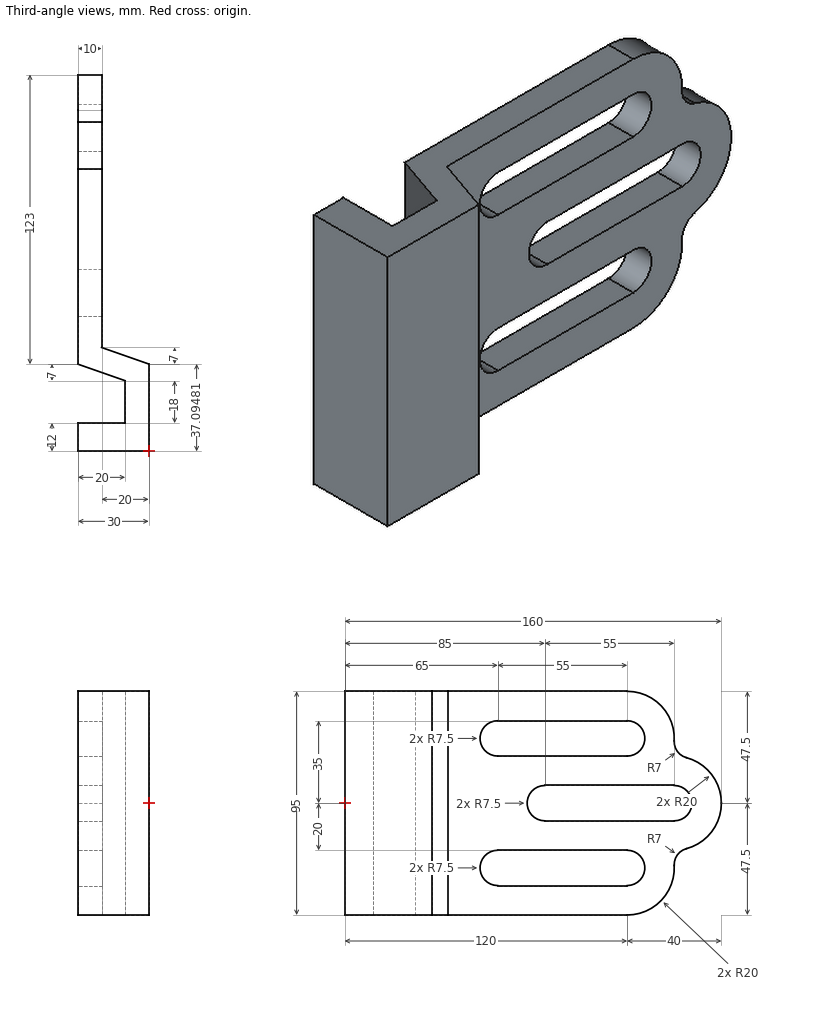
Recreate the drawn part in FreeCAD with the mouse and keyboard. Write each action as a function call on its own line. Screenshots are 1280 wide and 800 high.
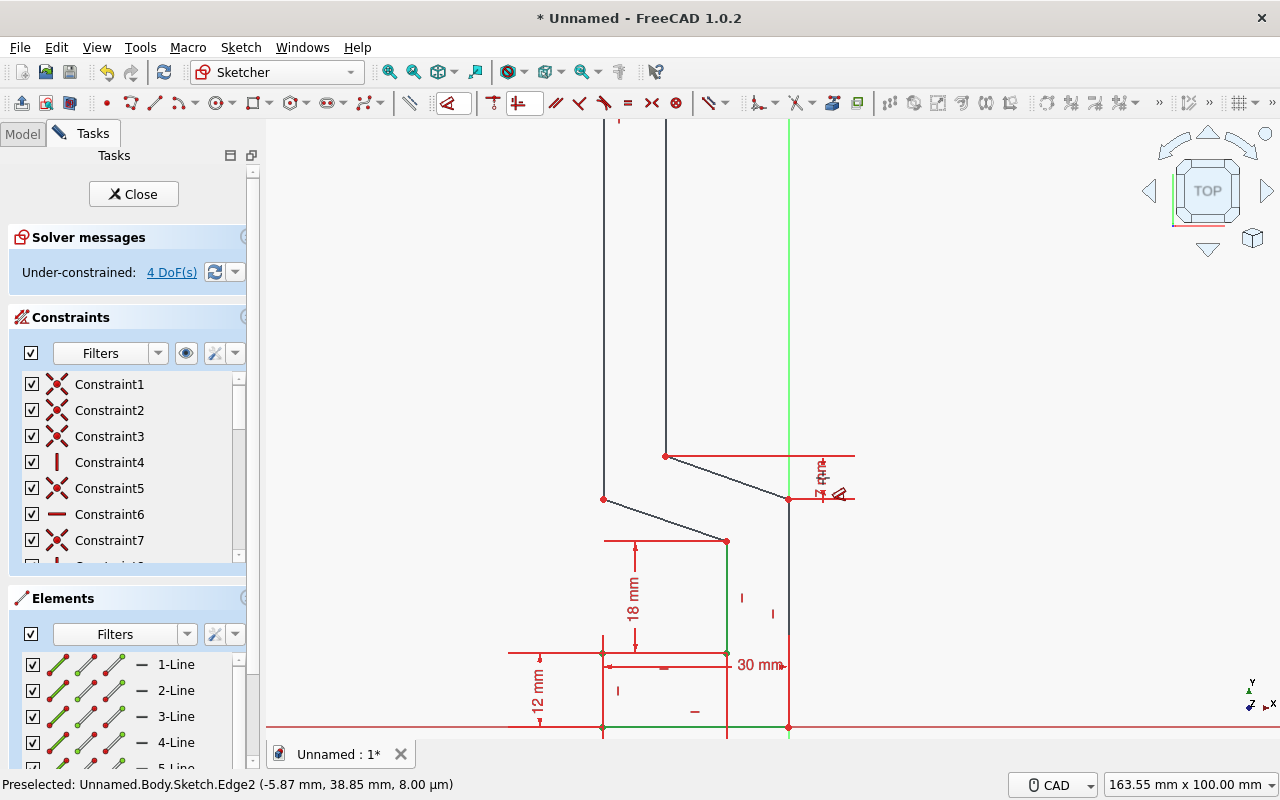
click(641, 512)
click(570, 520)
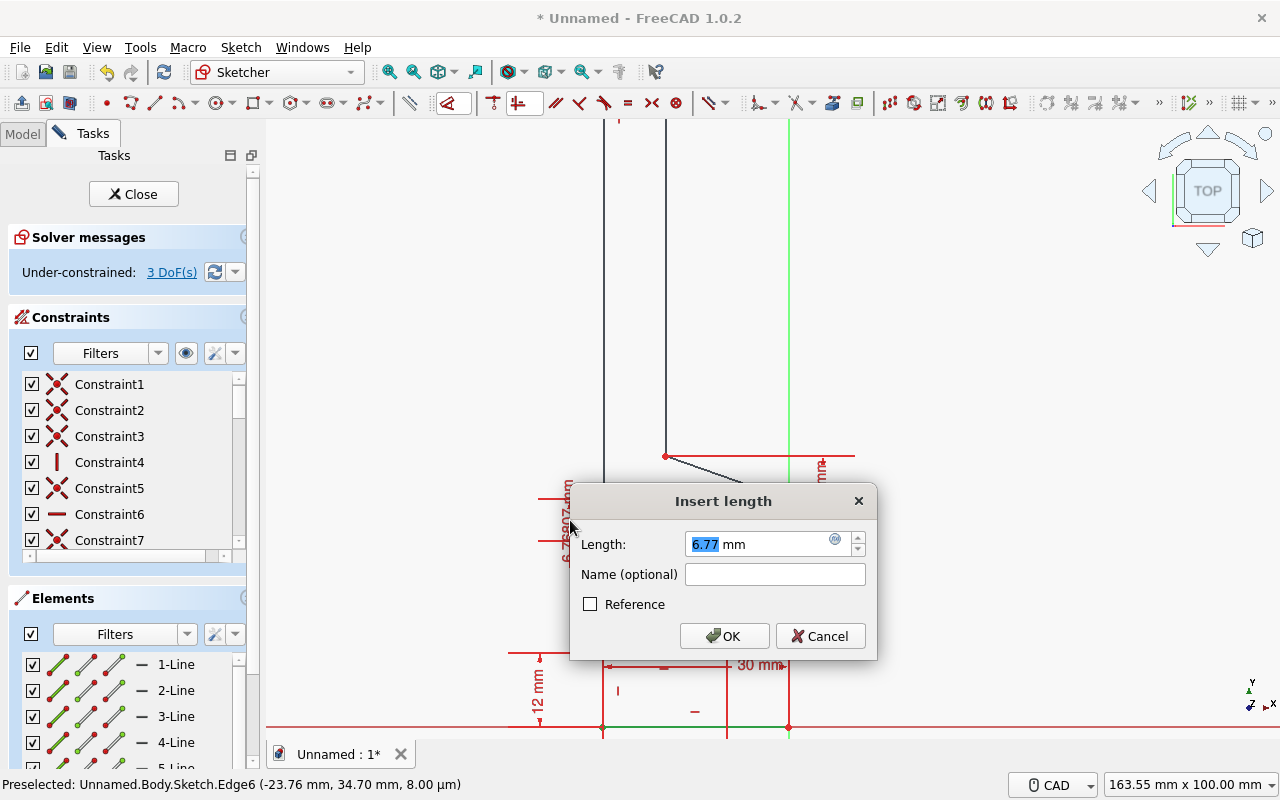
text(7)
key(Return)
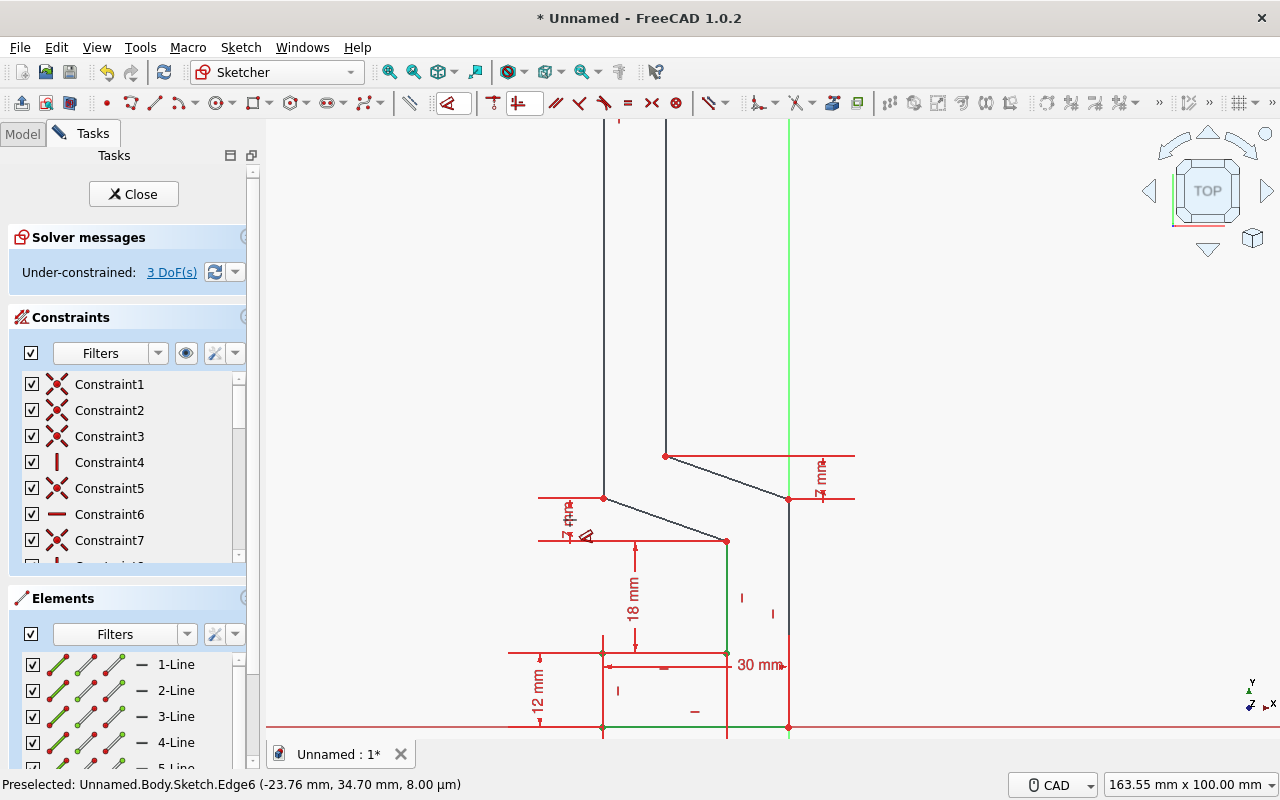
click(604, 270)
click(570, 323)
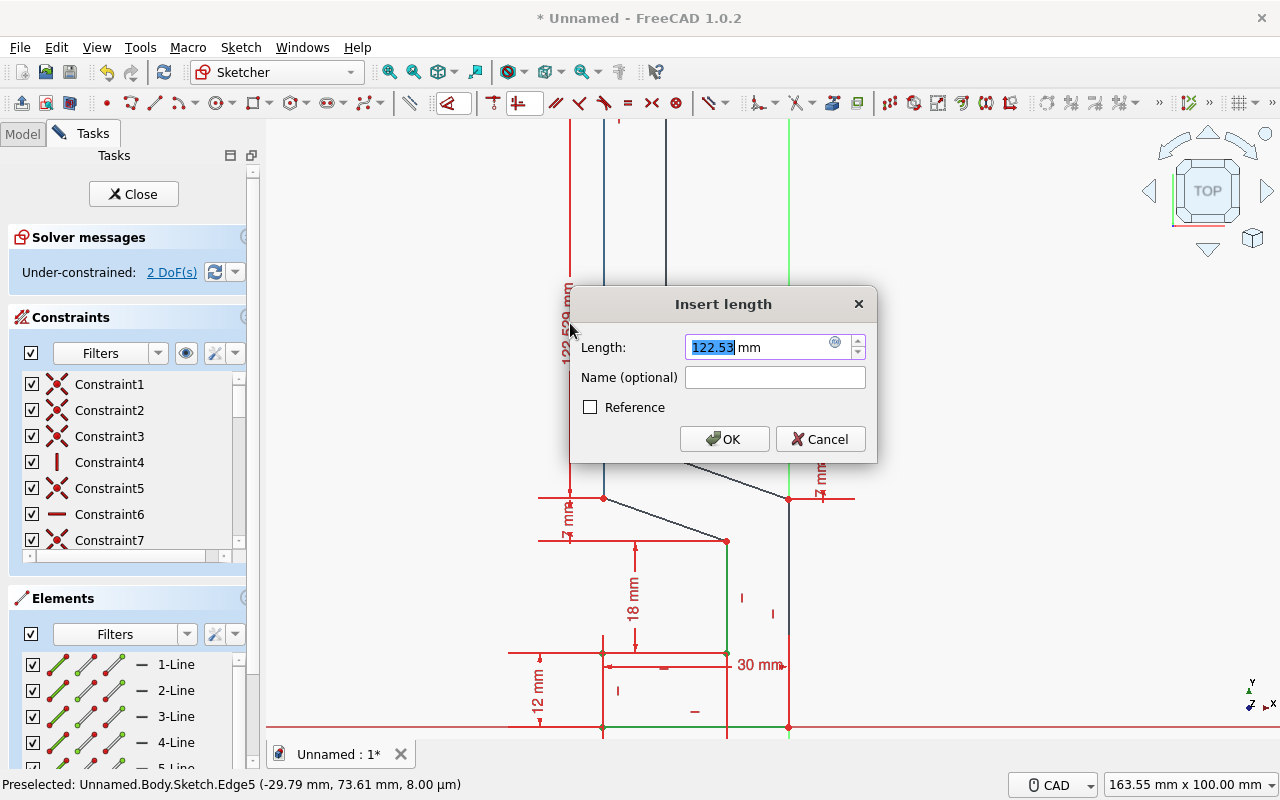
text(123)
key(Return)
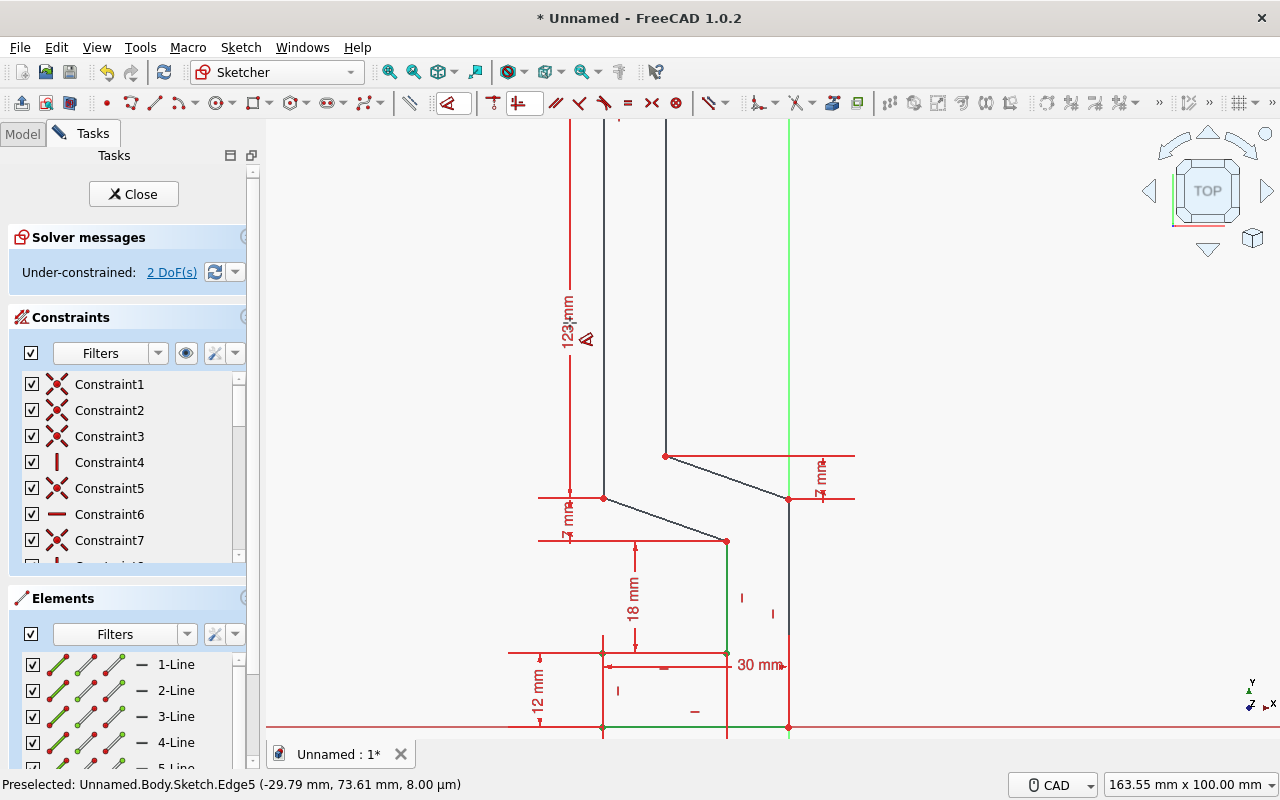
click(666, 456)
click(727, 422)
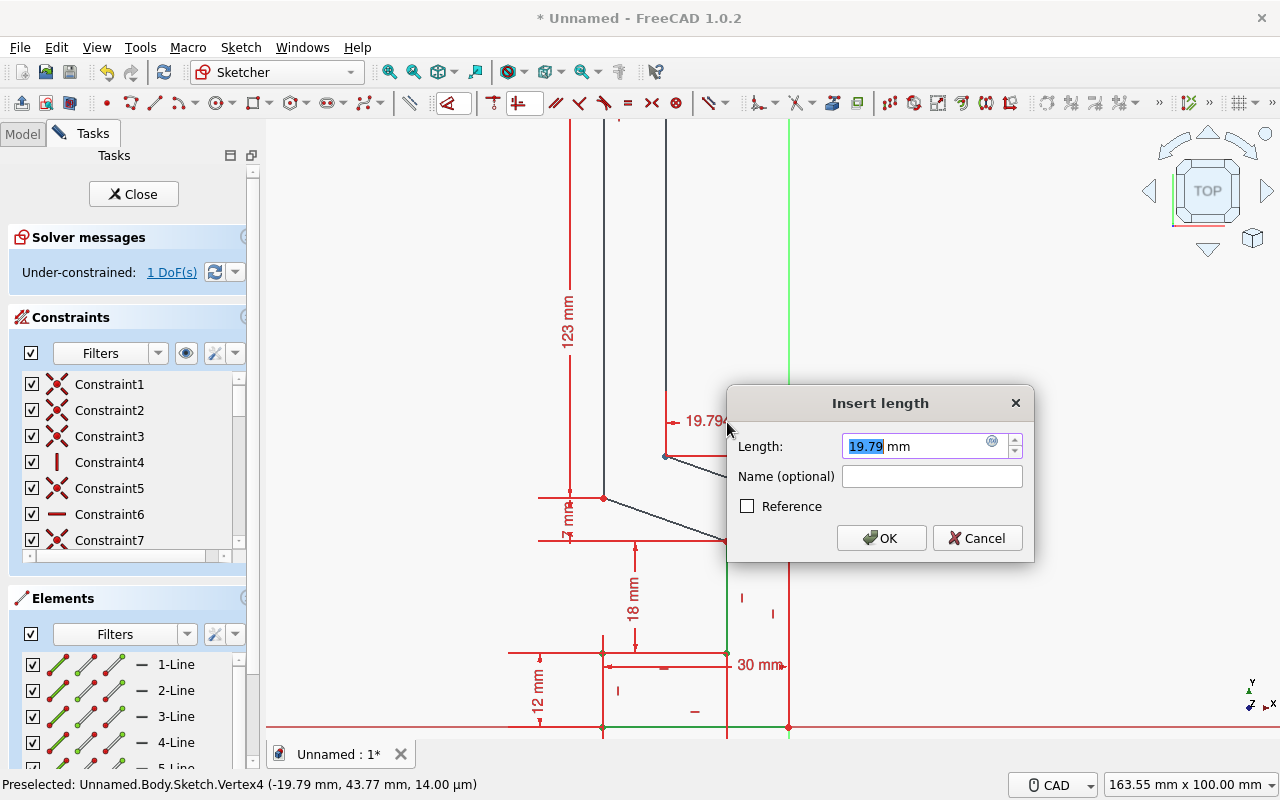
text(20)
key(Return)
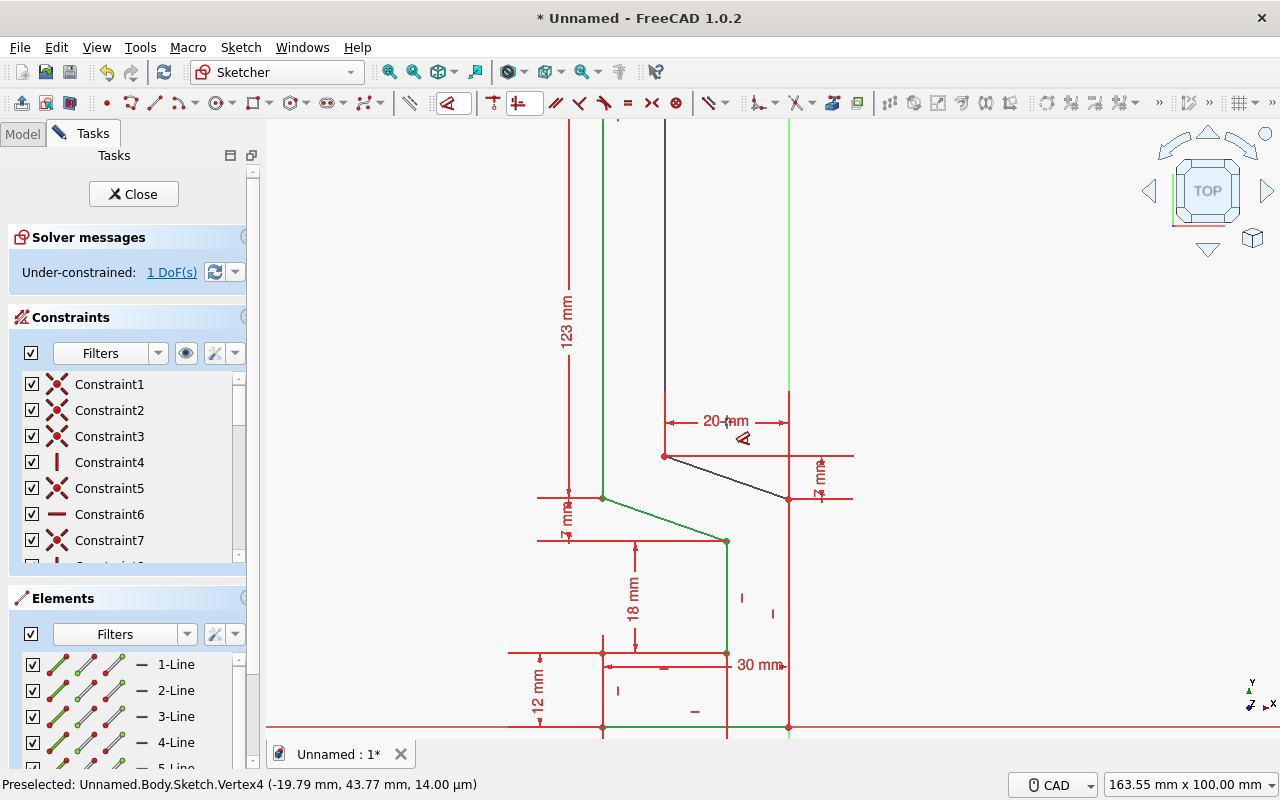
click(789, 659)
click(823, 605)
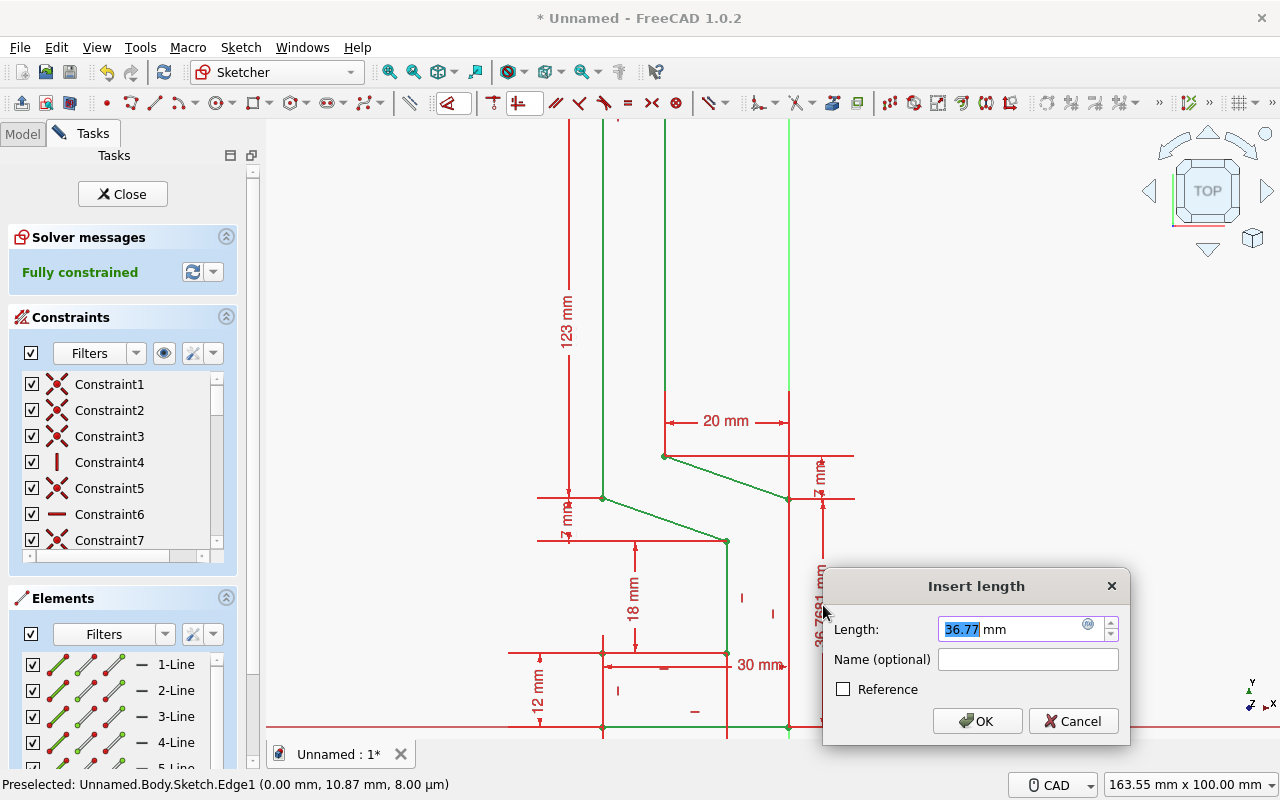
text(37.09481)
key(Return)
key(Escape)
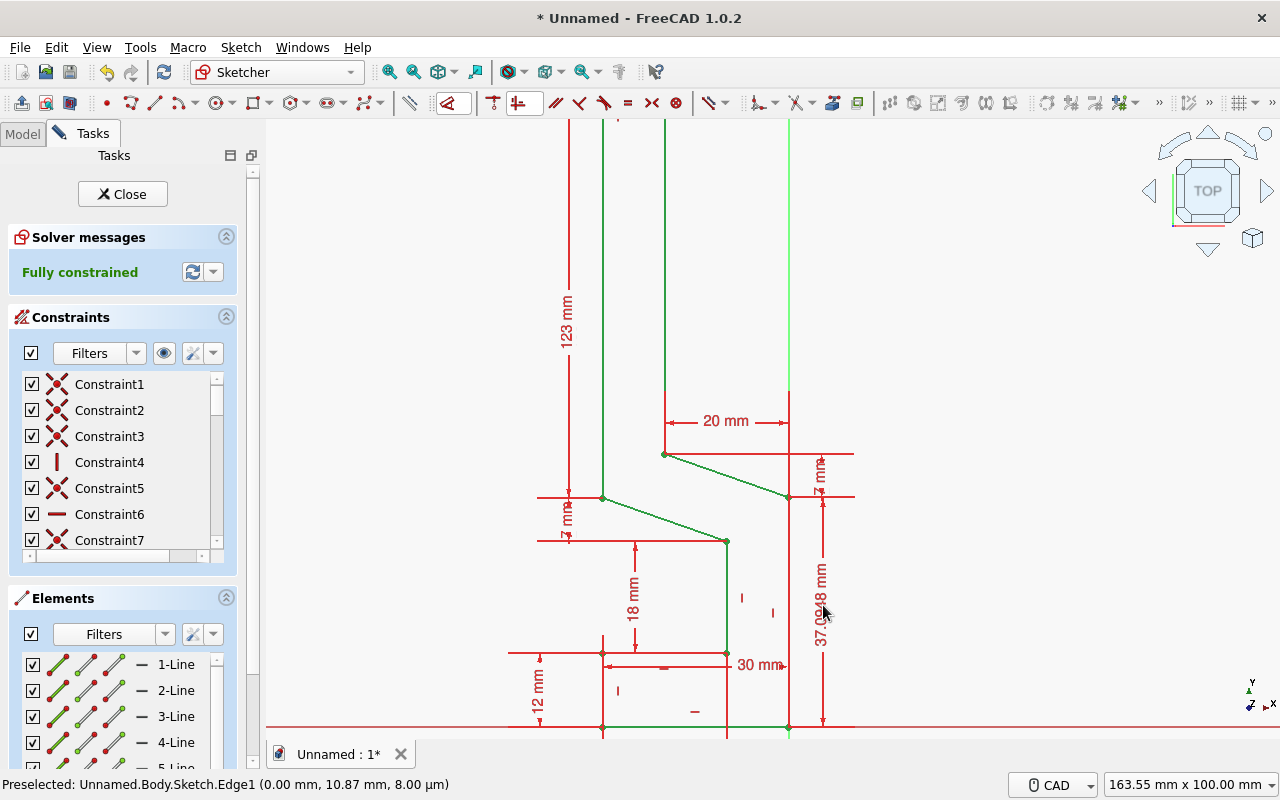
click(123, 194)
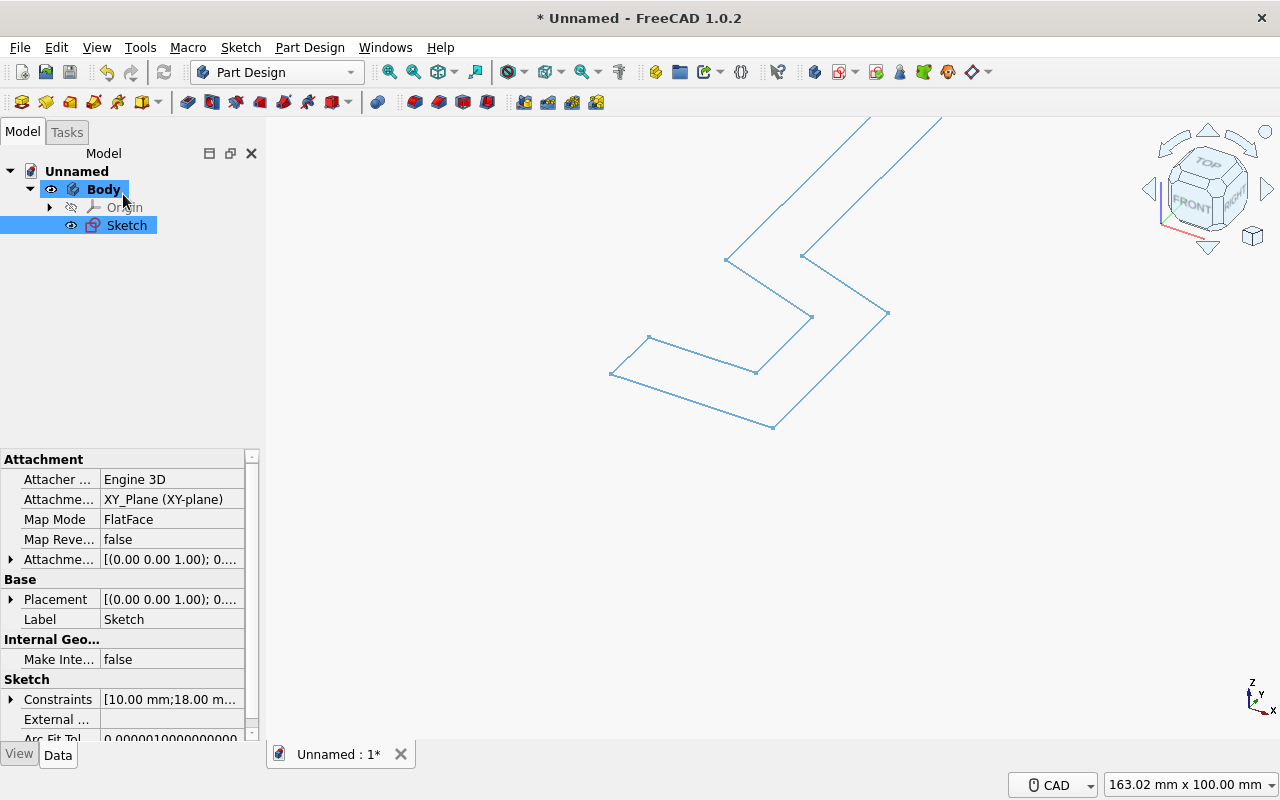
click(22, 102)